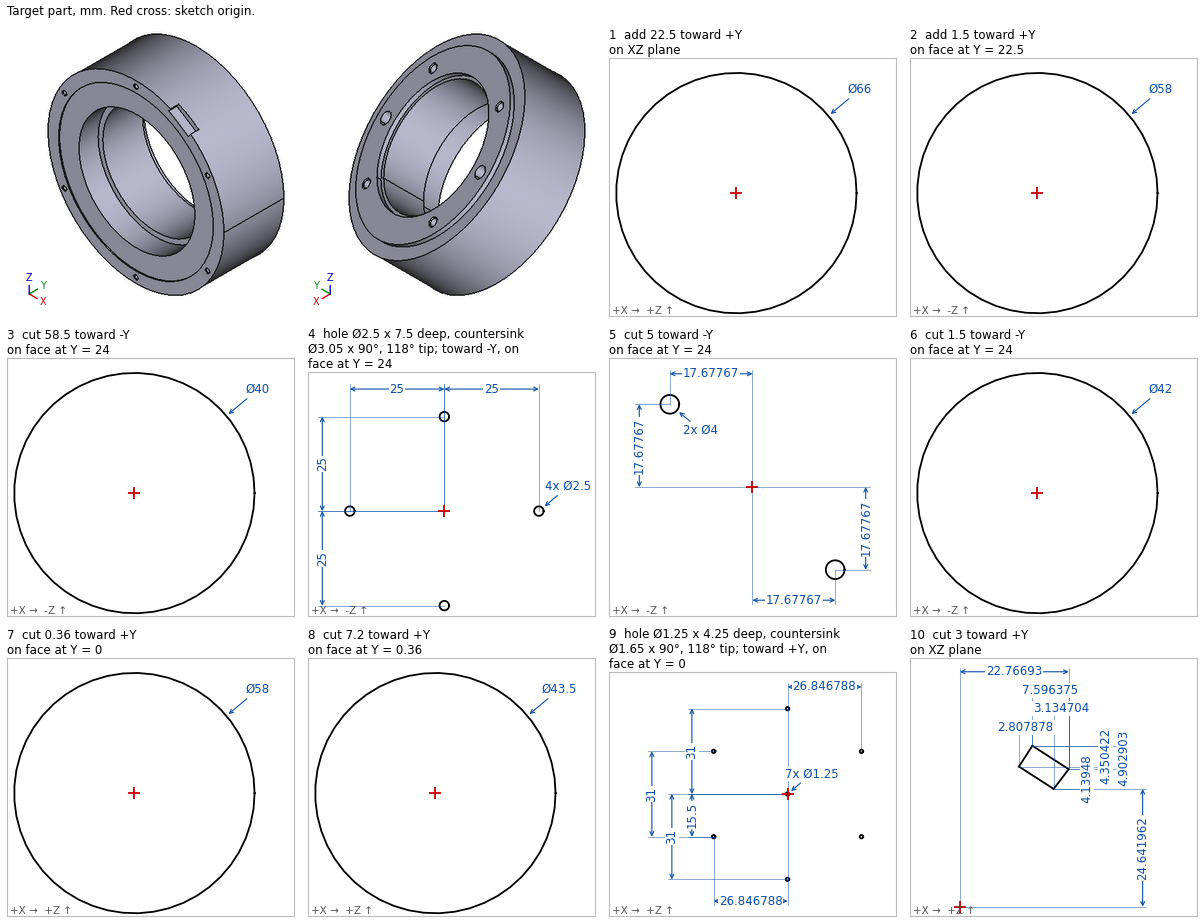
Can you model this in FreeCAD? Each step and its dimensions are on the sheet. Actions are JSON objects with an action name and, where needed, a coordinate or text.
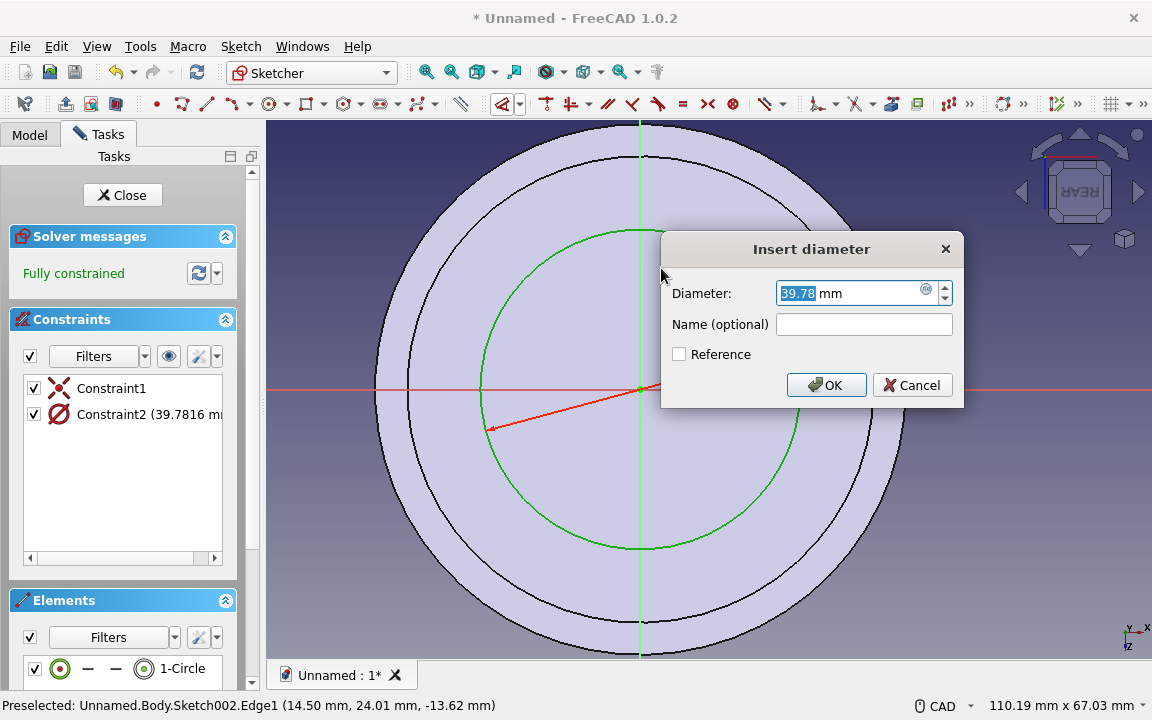
{"action": "type", "text": "40"}
{"action": "key", "text": "Return"}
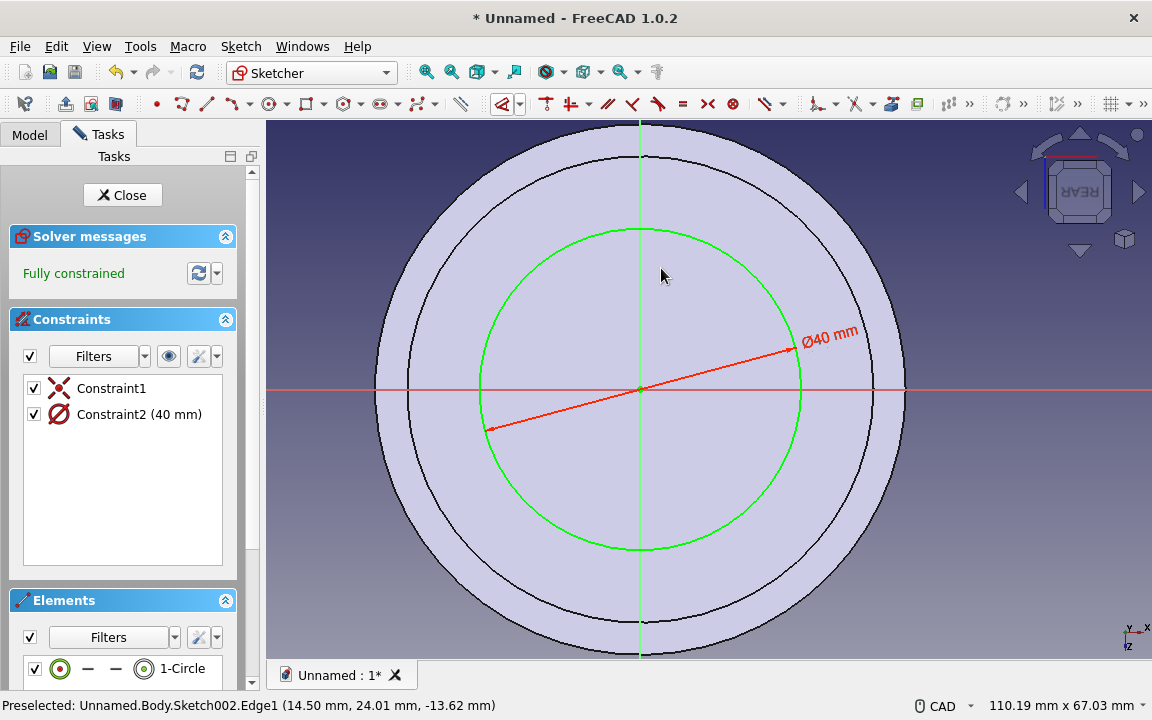
{"action": "left_click", "coordinate": [123, 195]}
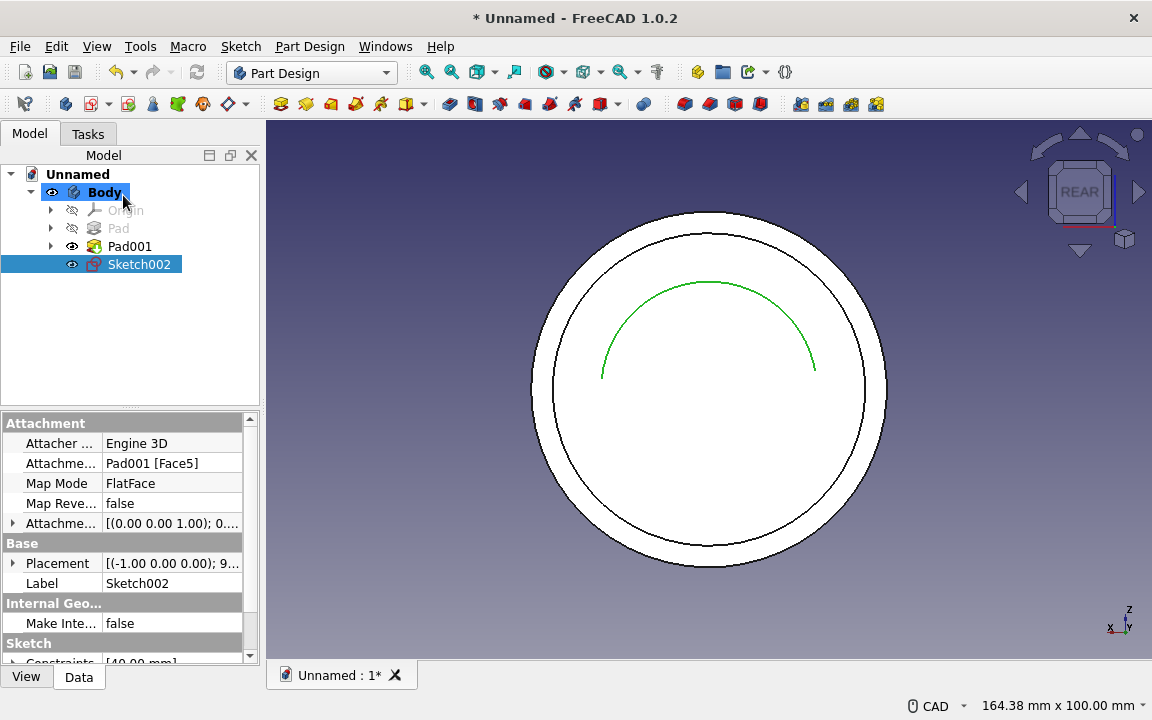
{"action": "left_click", "coordinate": [450, 104]}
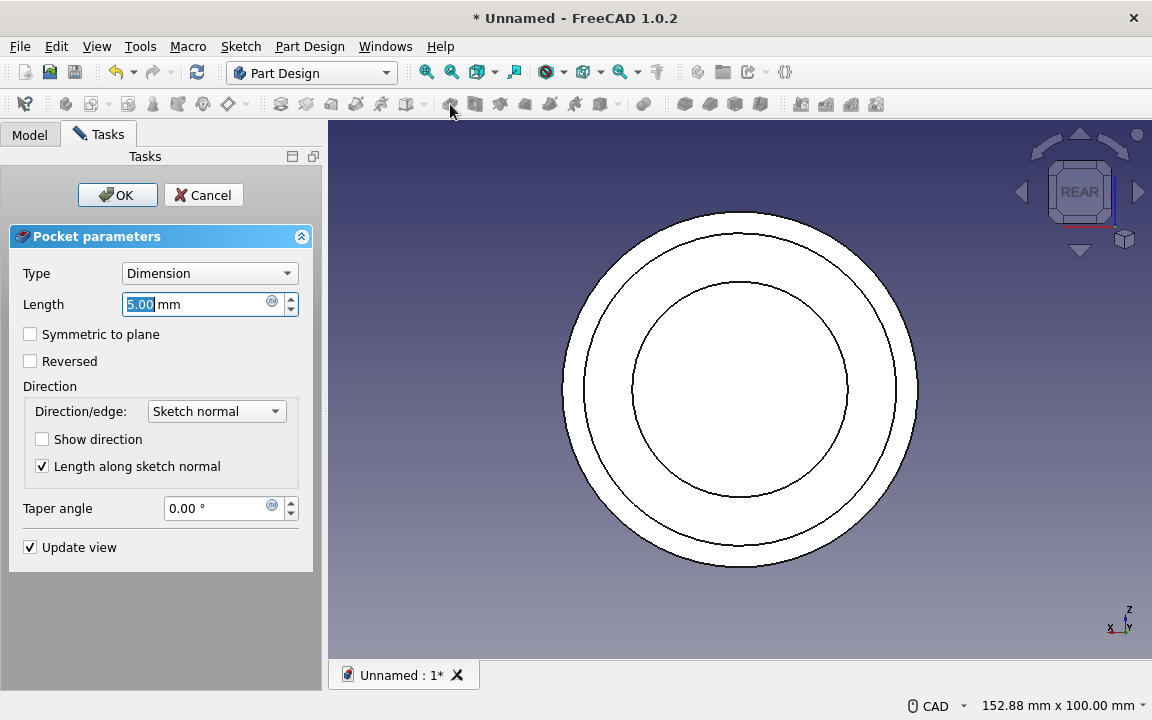
{"action": "type", "text": "58.5"}
{"action": "key", "text": "Tab"}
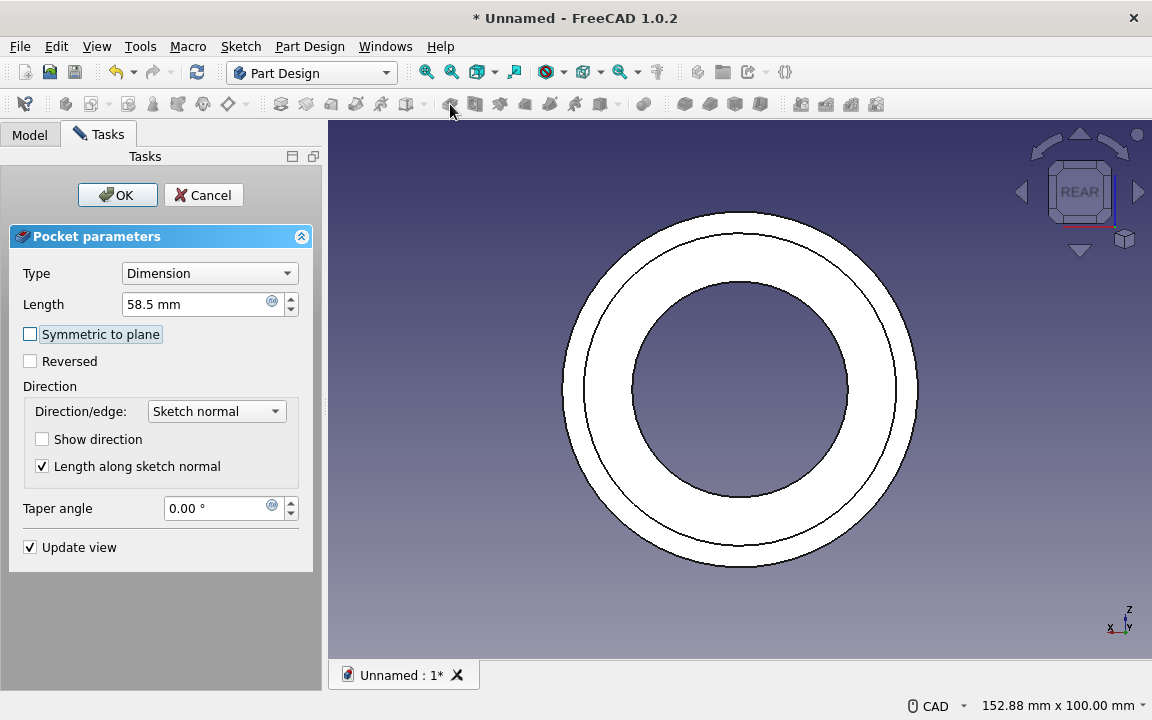
{"action": "left_click", "coordinate": [118, 195]}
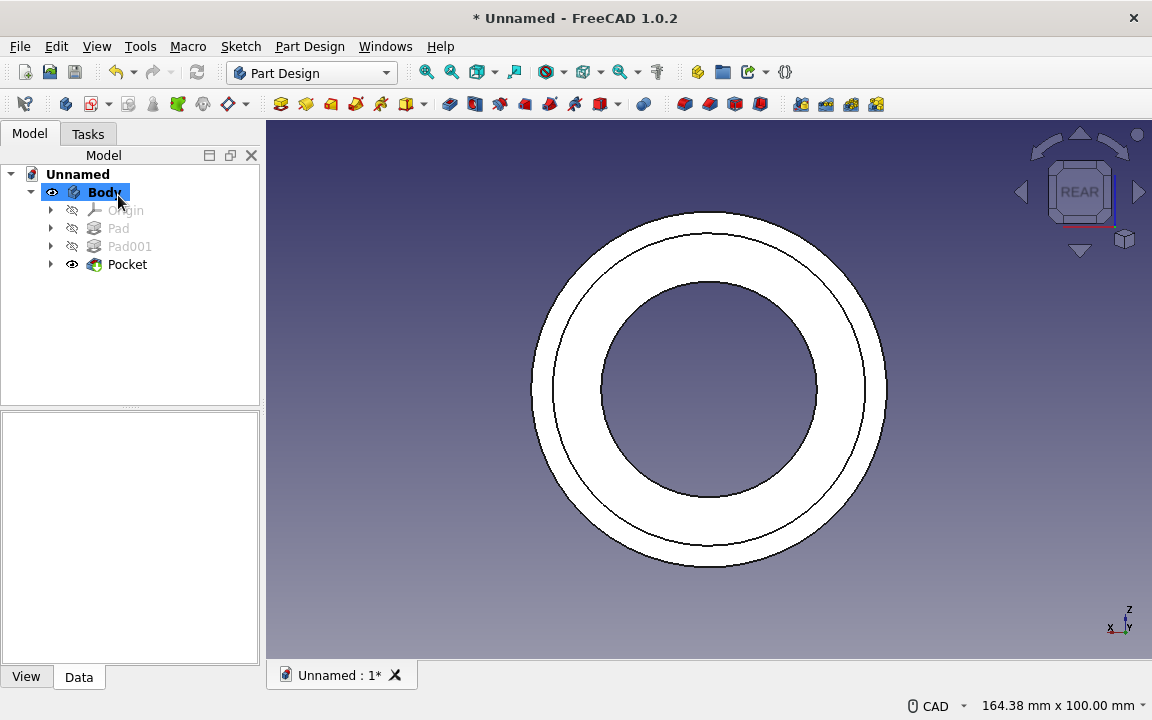
{"action": "left_click", "coordinate": [575, 388]}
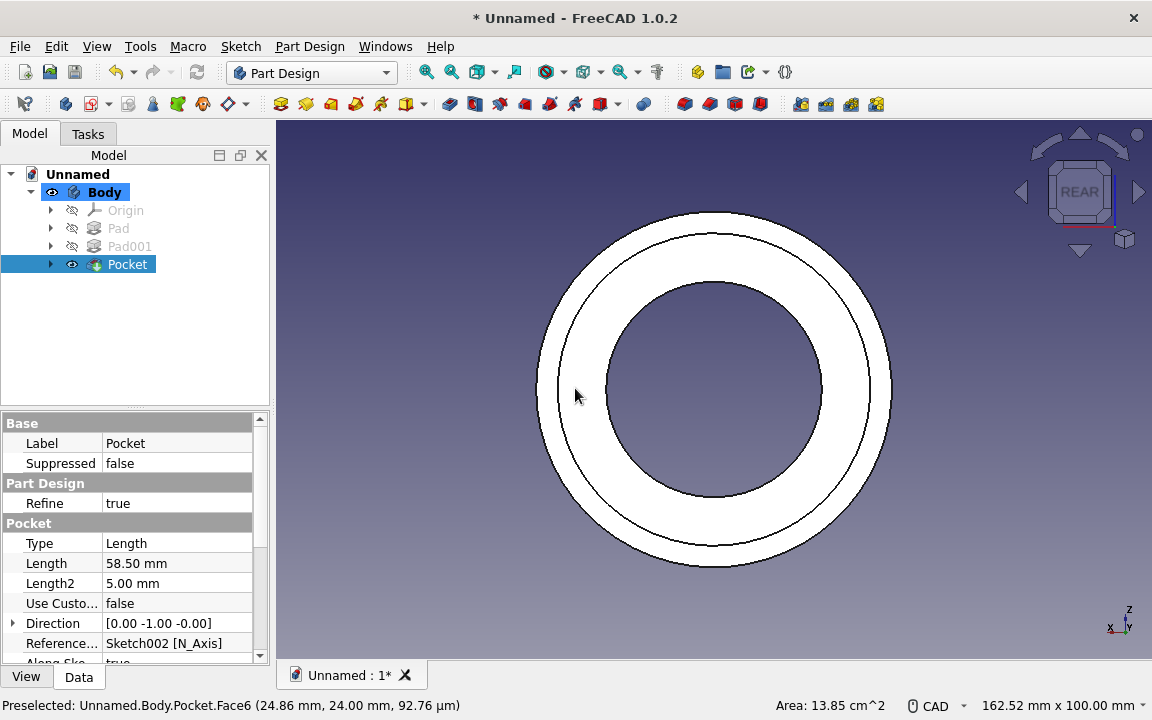
{"action": "left_click", "coordinate": [90, 104]}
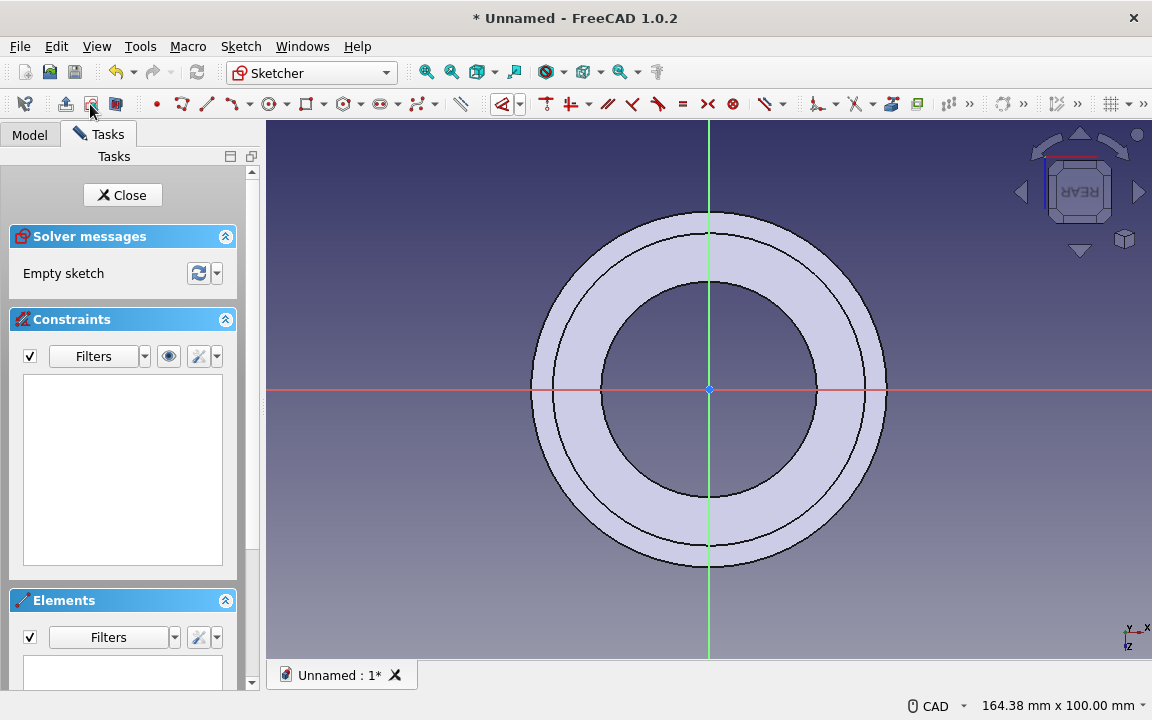
{"action": "left_click", "coordinate": [268, 104]}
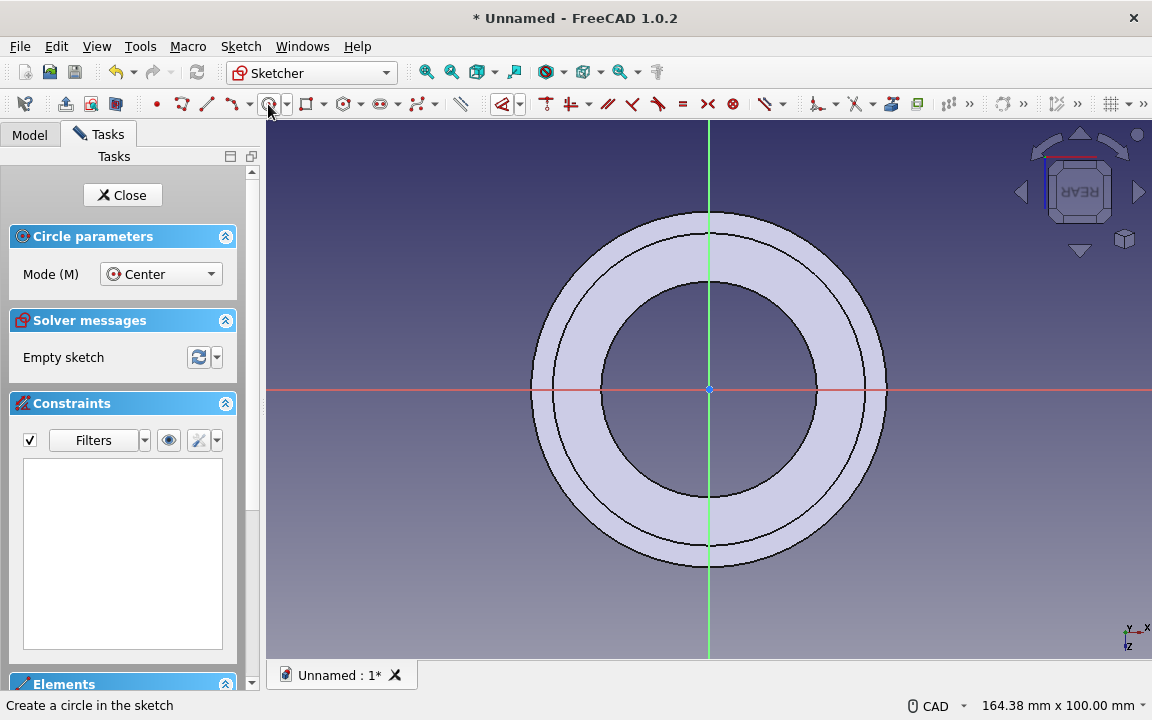
{"action": "scroll", "coordinate": [844, 389], "scroll_direction": "up", "scroll_amount": 7}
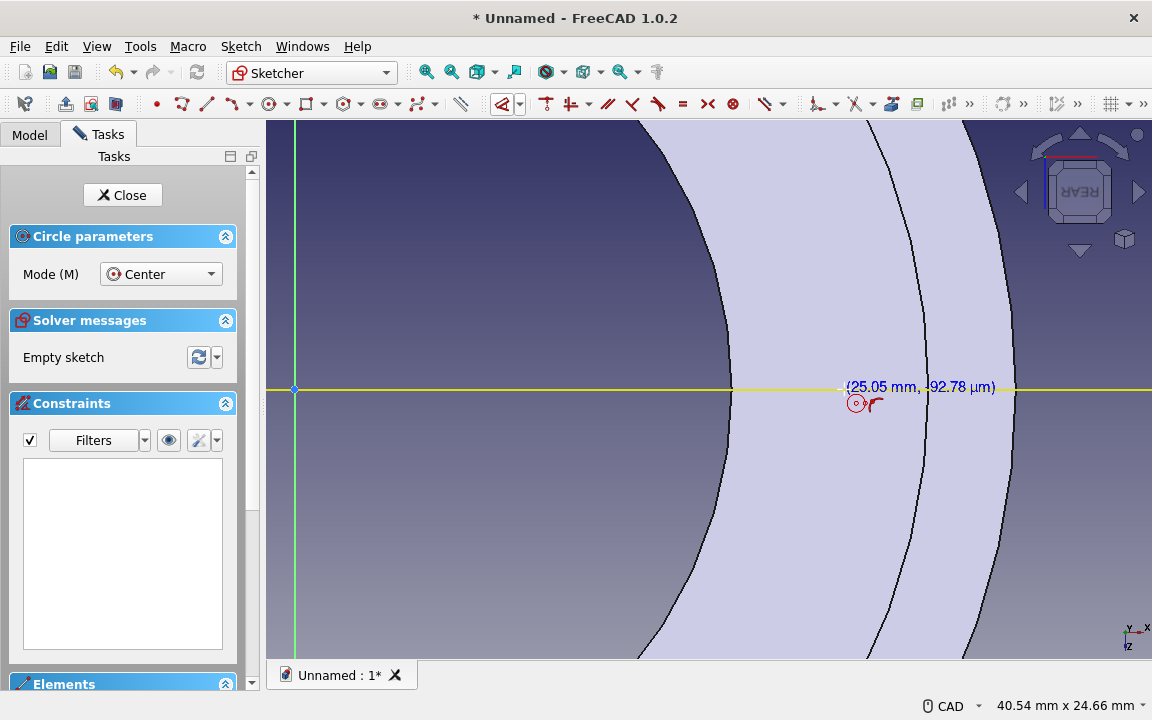
{"action": "scroll", "coordinate": [790, 390], "scroll_direction": "down", "scroll_amount": 6}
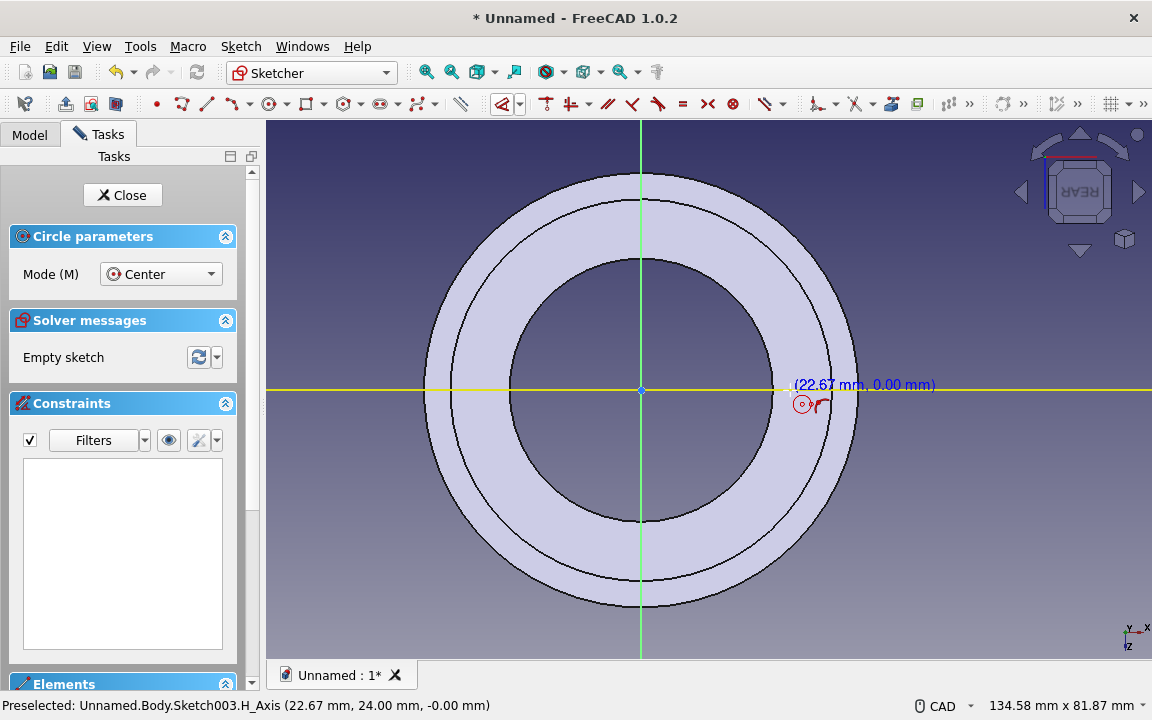
{"action": "left_click", "coordinate": [806, 390]}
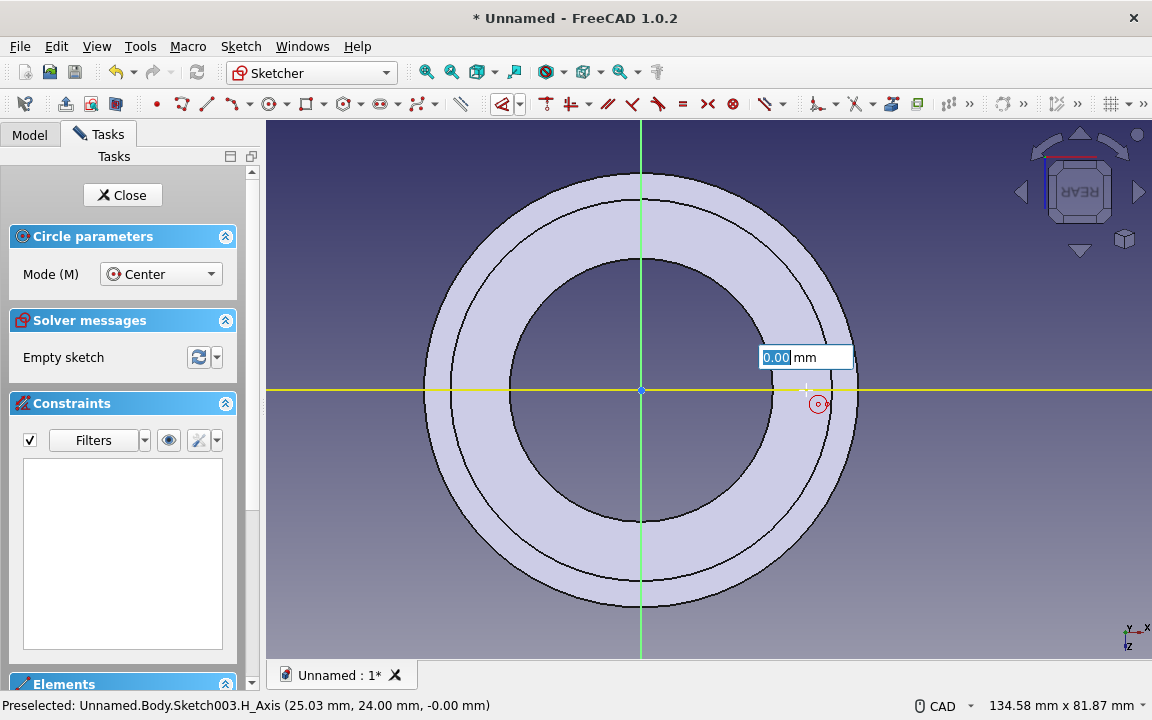
{"action": "scroll", "coordinate": [803, 398], "scroll_direction": "up", "scroll_amount": 4}